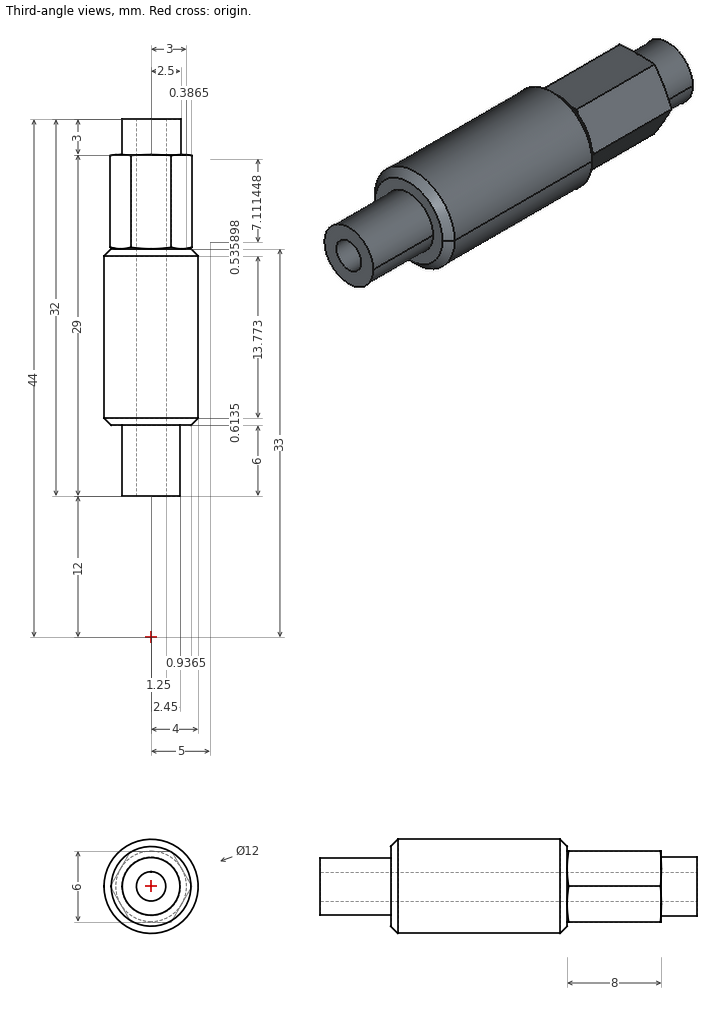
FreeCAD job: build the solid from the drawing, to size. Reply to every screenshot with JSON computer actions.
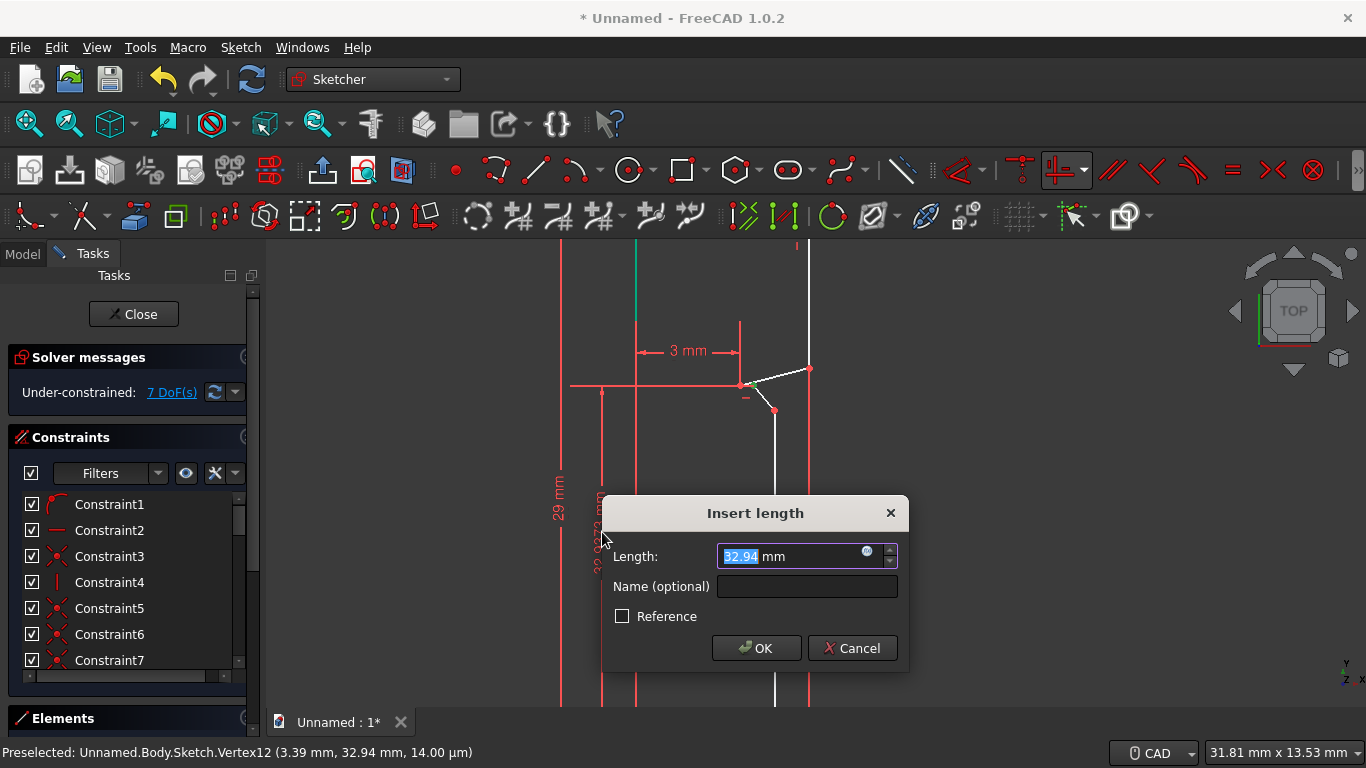
{"action": "type", "text": "33"}
{"action": "key", "text": "Return"}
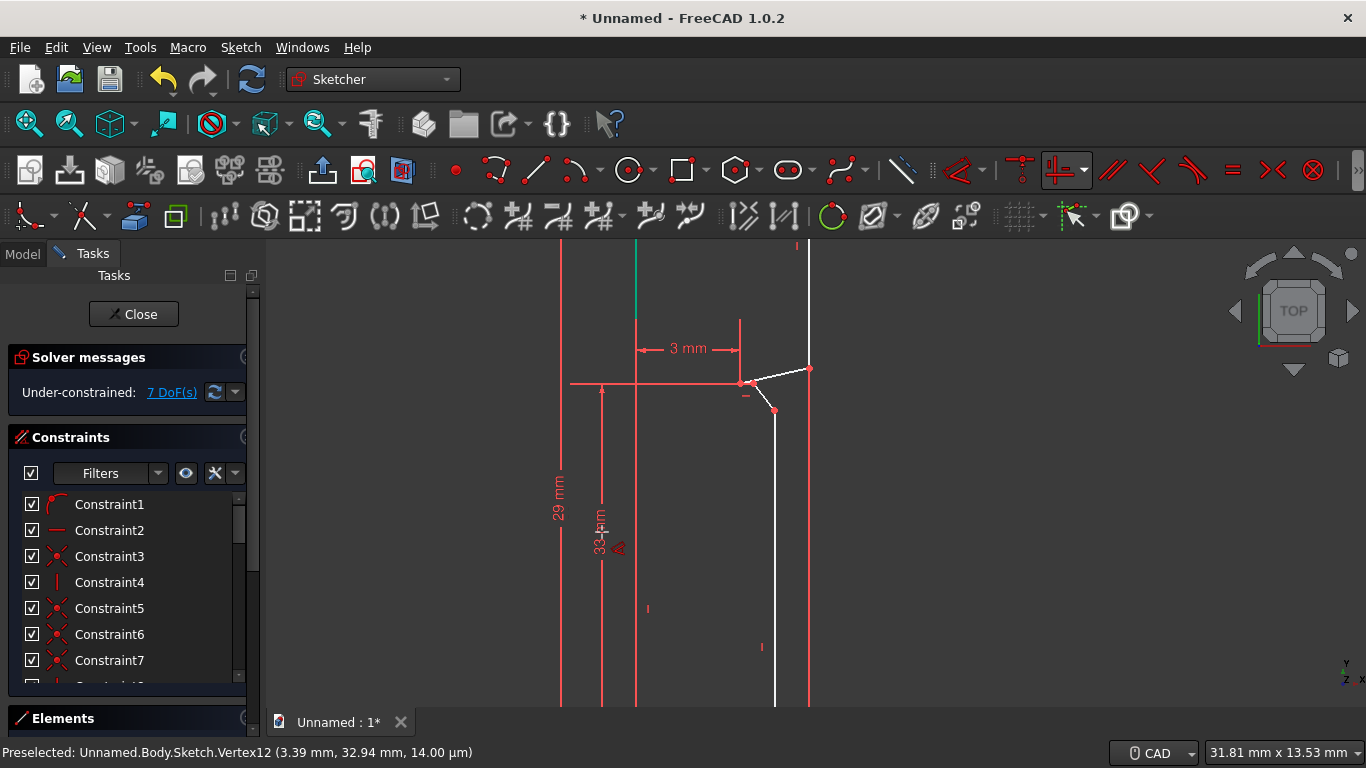
{"action": "scroll", "coordinate": [754, 386], "scroll_direction": "down", "scroll_amount": 8}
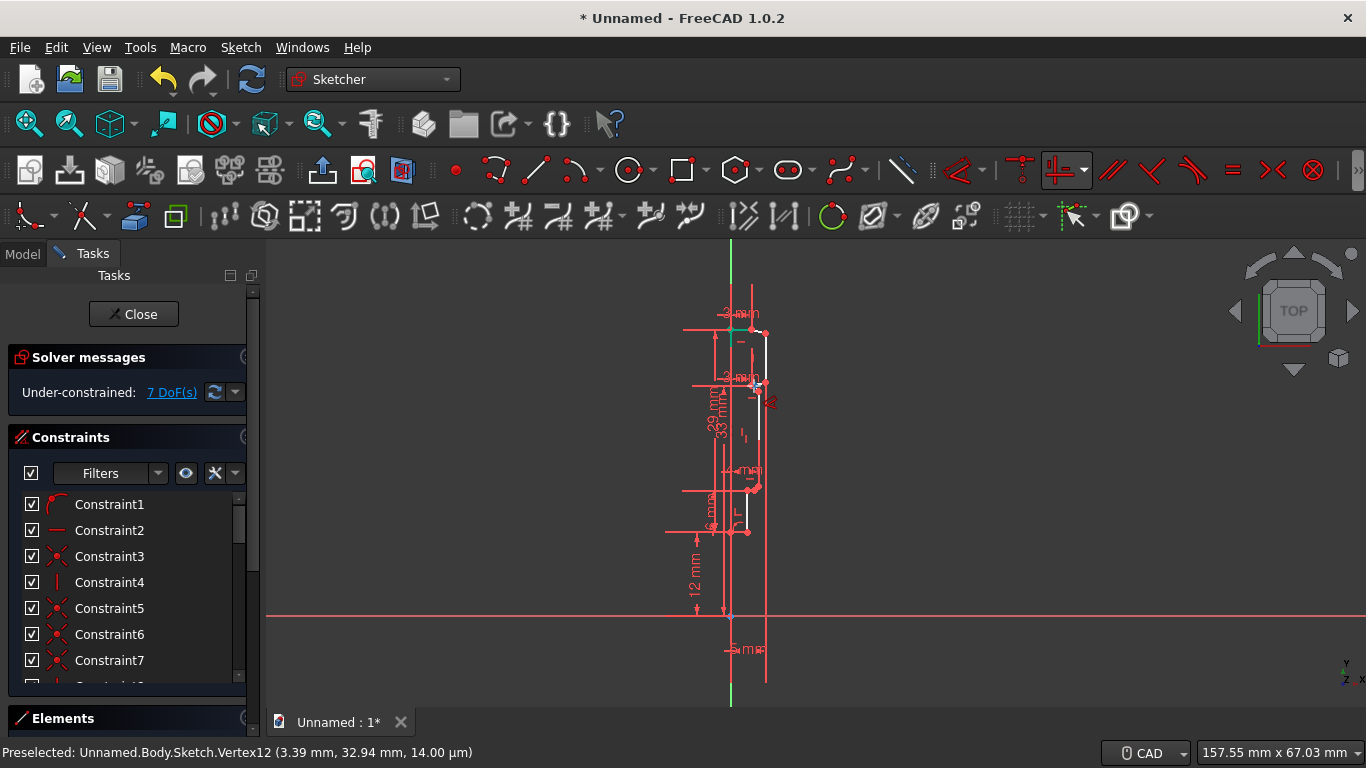
{"action": "scroll", "coordinate": [736, 532], "scroll_direction": "up", "scroll_amount": 6}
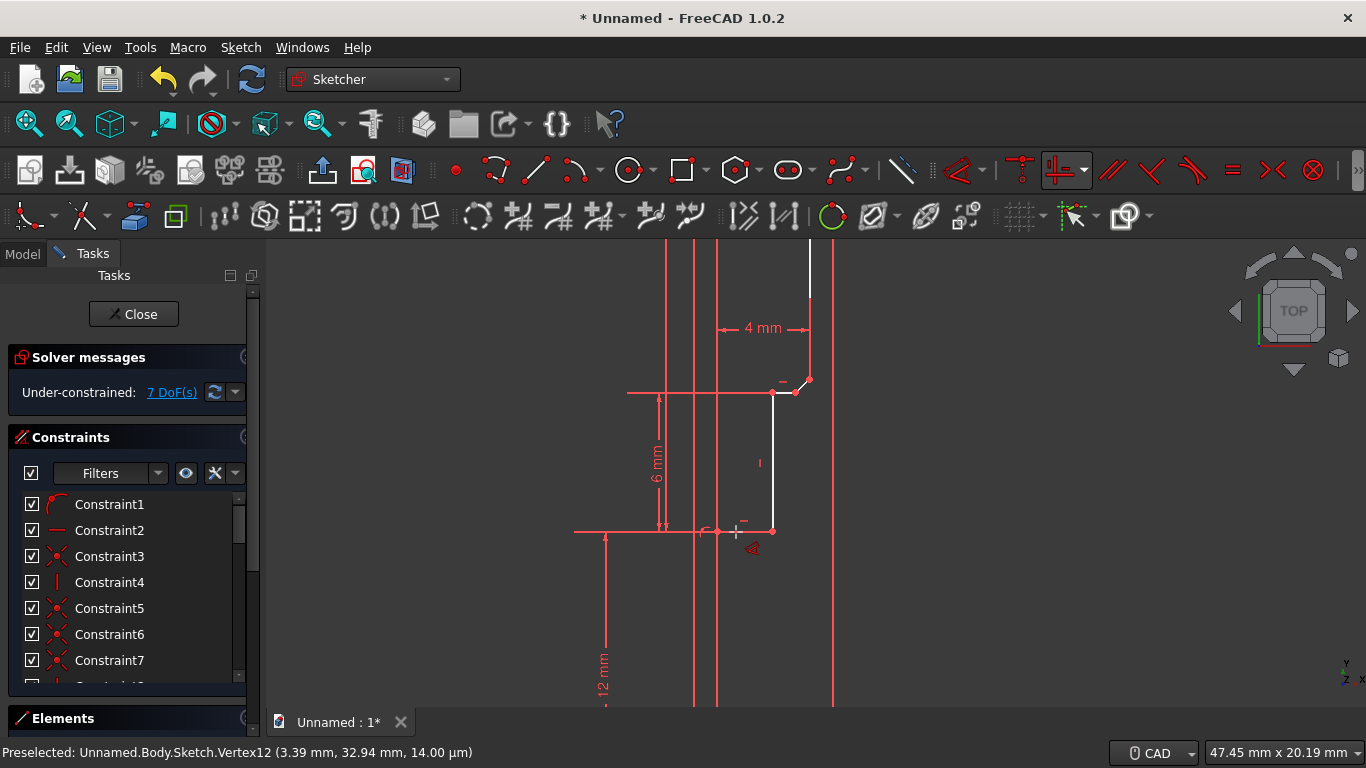
{"action": "left_click", "coordinate": [734, 532]}
{"action": "left_click", "coordinate": [745, 566]}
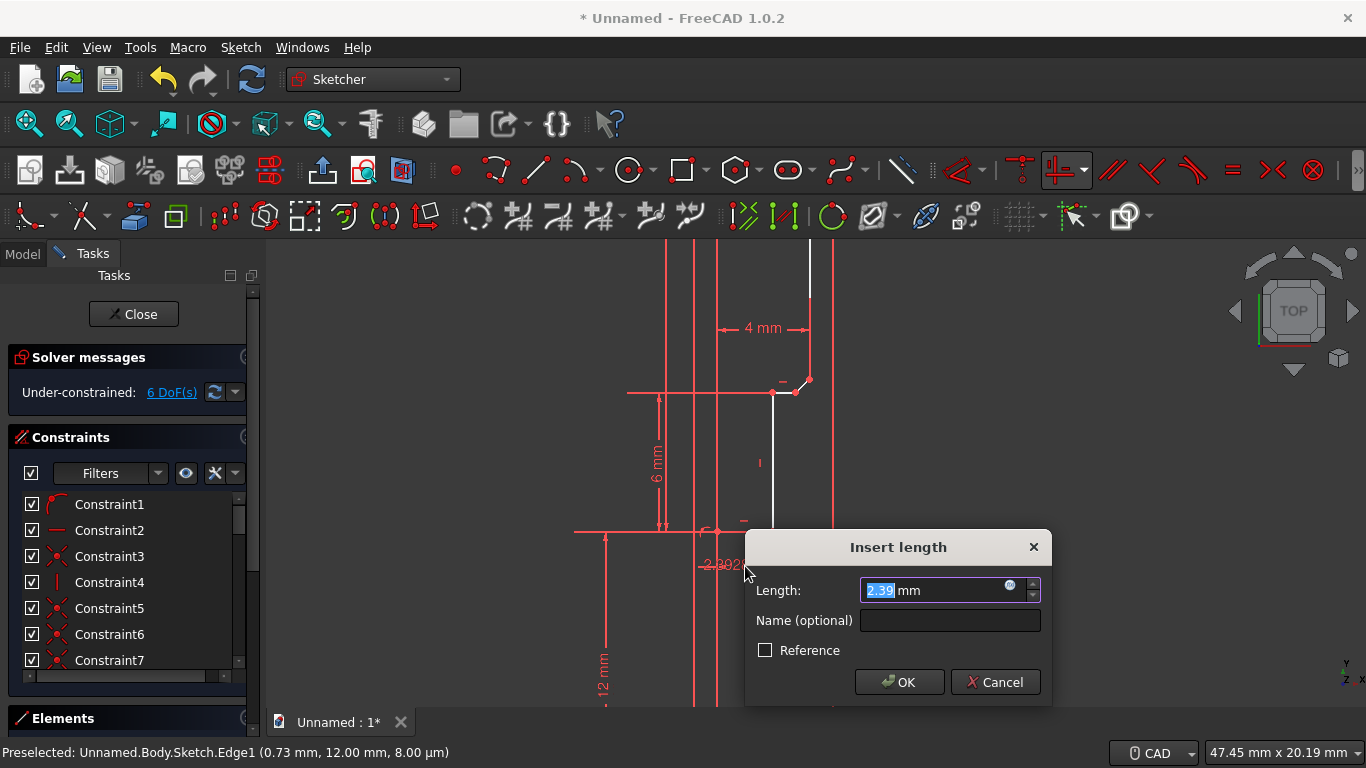
{"action": "type", "text": "2.45"}
{"action": "key", "text": "Return"}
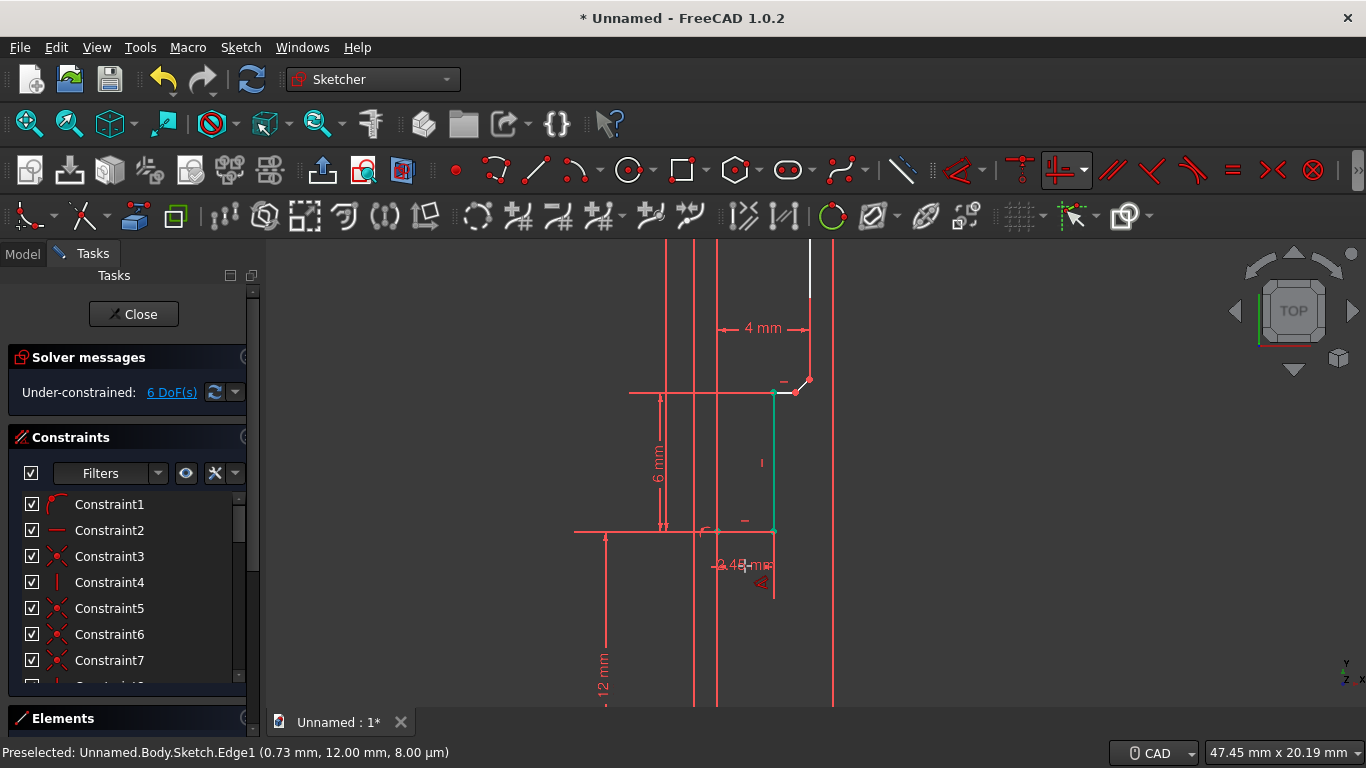
{"action": "scroll", "coordinate": [785, 393], "scroll_direction": "up", "scroll_amount": 4}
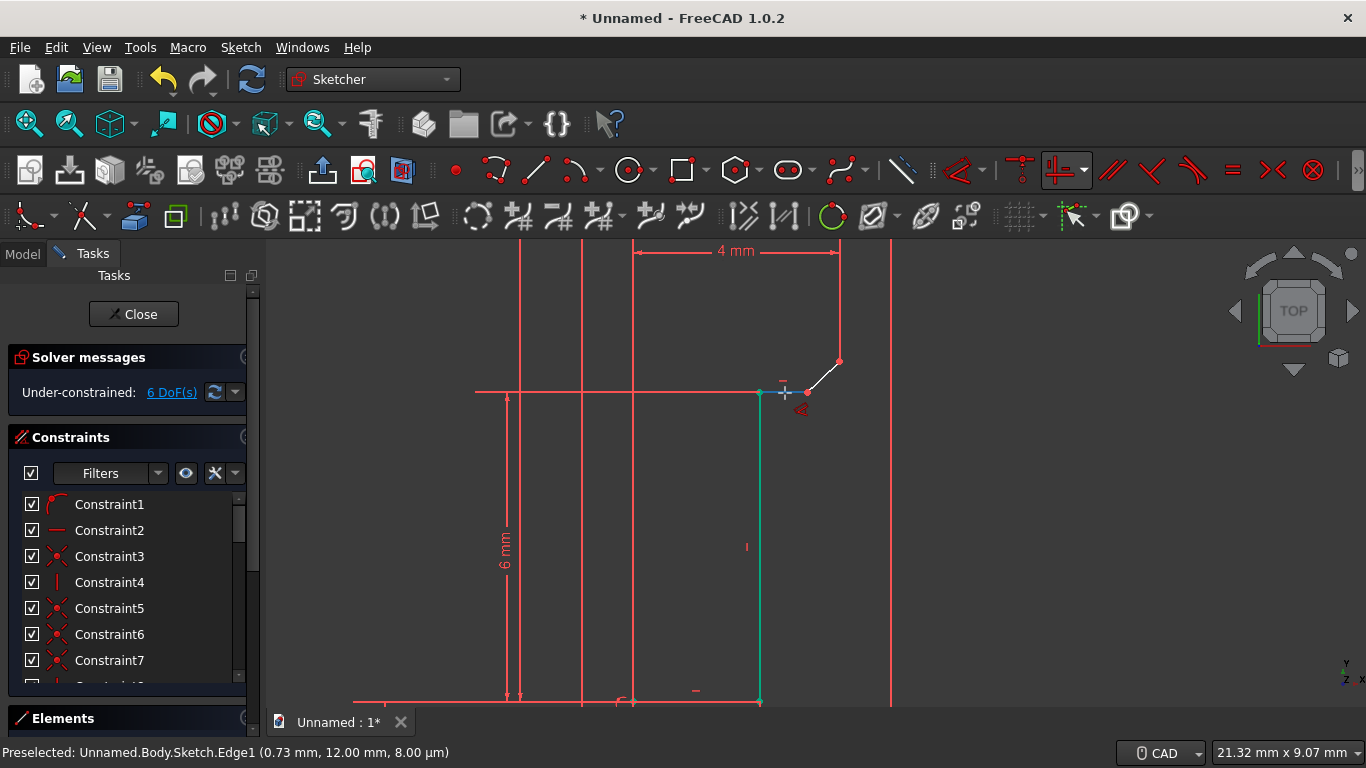
{"action": "left_click", "coordinate": [784, 392]}
{"action": "left_click", "coordinate": [784, 426]}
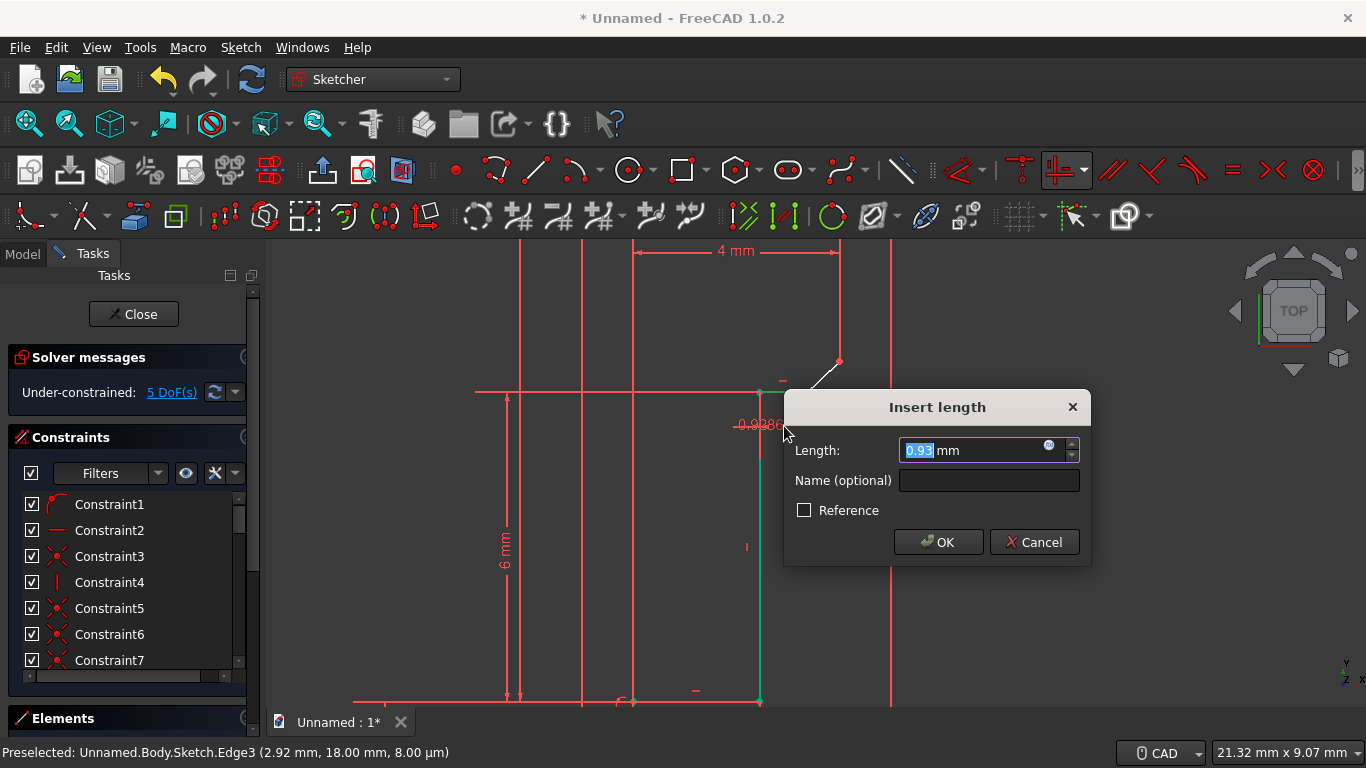
{"action": "type", "text": "0.9365"}
{"action": "key", "text": "Return"}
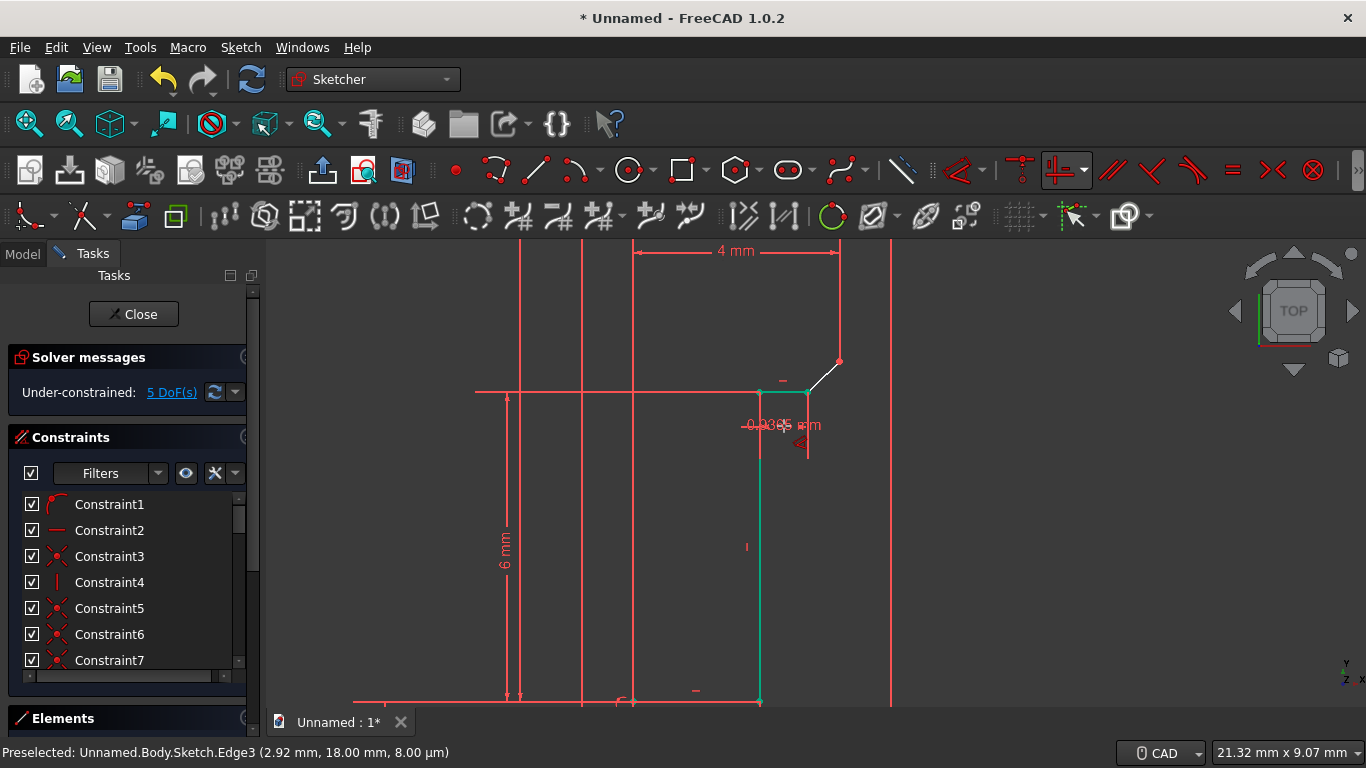
{"action": "scroll", "coordinate": [745, 506], "scroll_direction": "down", "scroll_amount": 10}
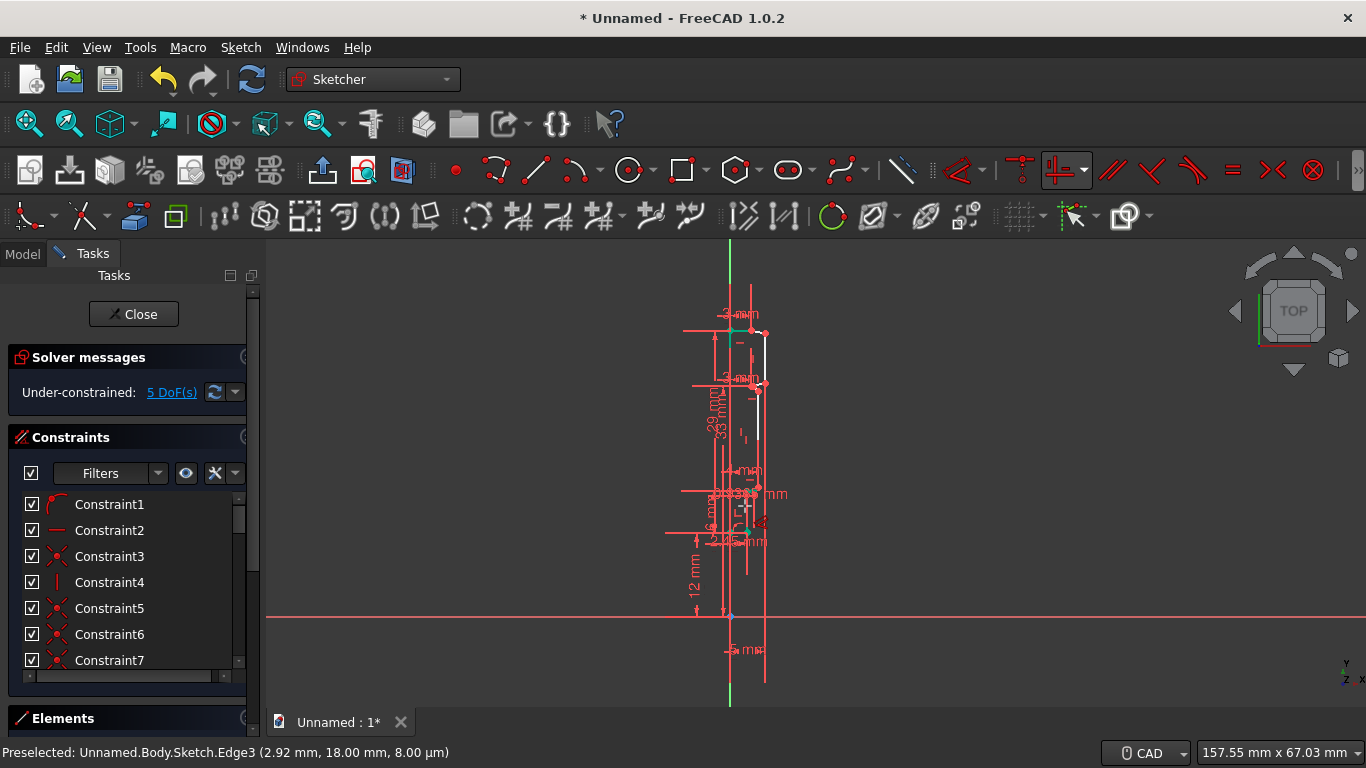
{"action": "left_click", "coordinate": [758, 458]}
{"action": "left_click", "coordinate": [792, 439]}